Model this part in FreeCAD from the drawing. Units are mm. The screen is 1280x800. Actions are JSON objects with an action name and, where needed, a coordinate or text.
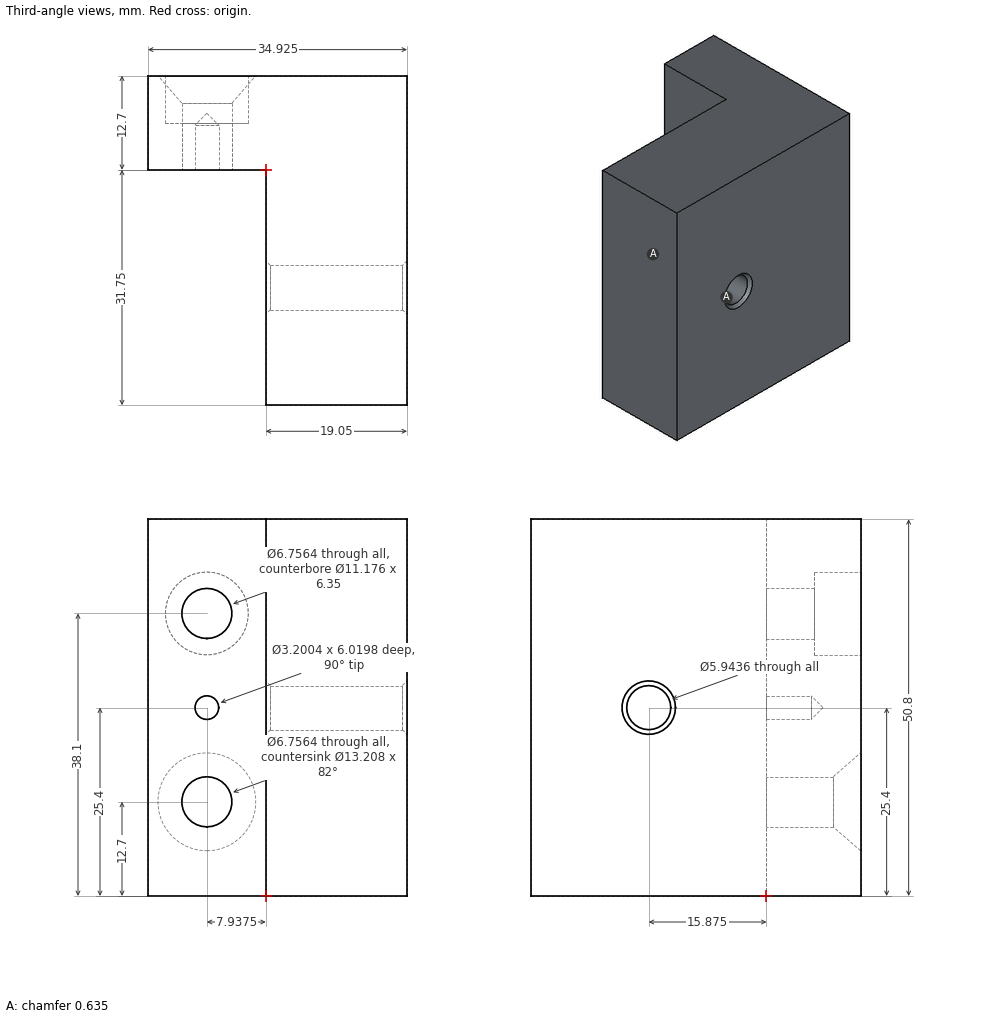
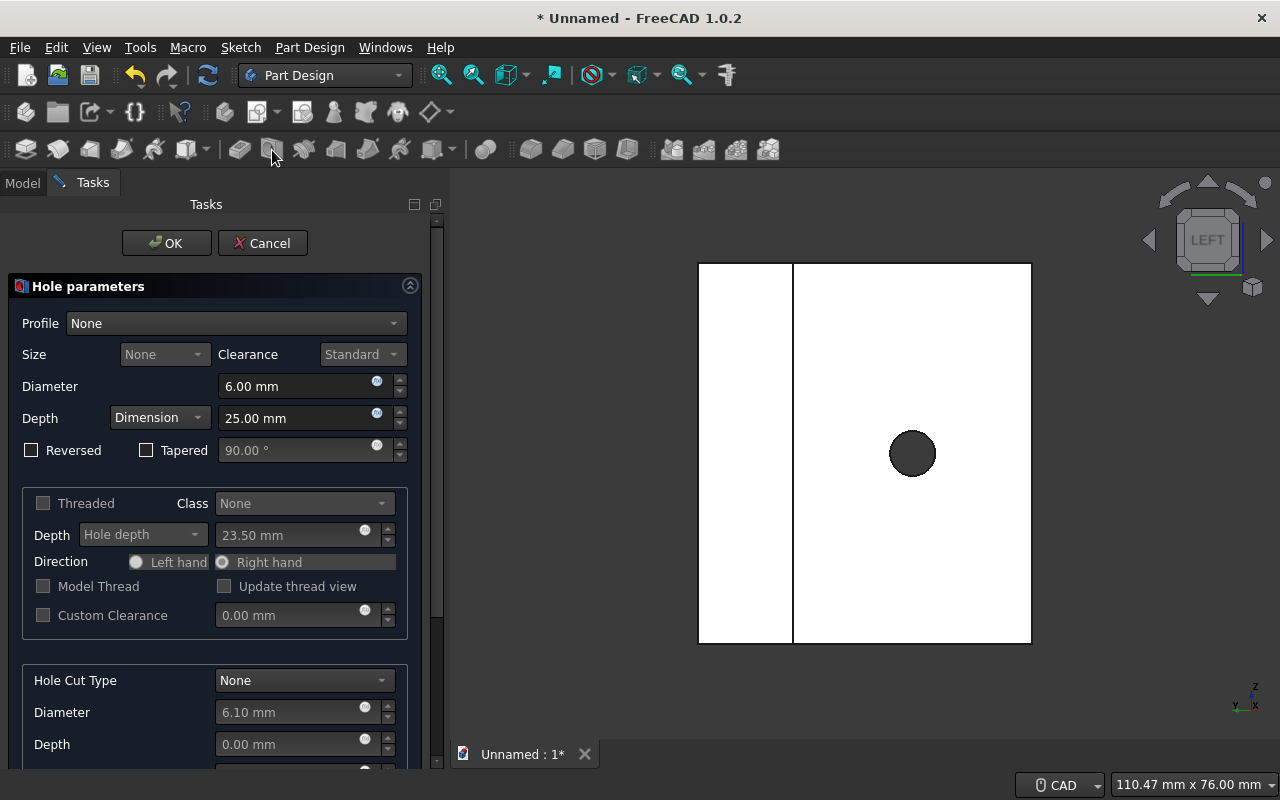
{"action": "triple_click", "coordinate": [305, 386]}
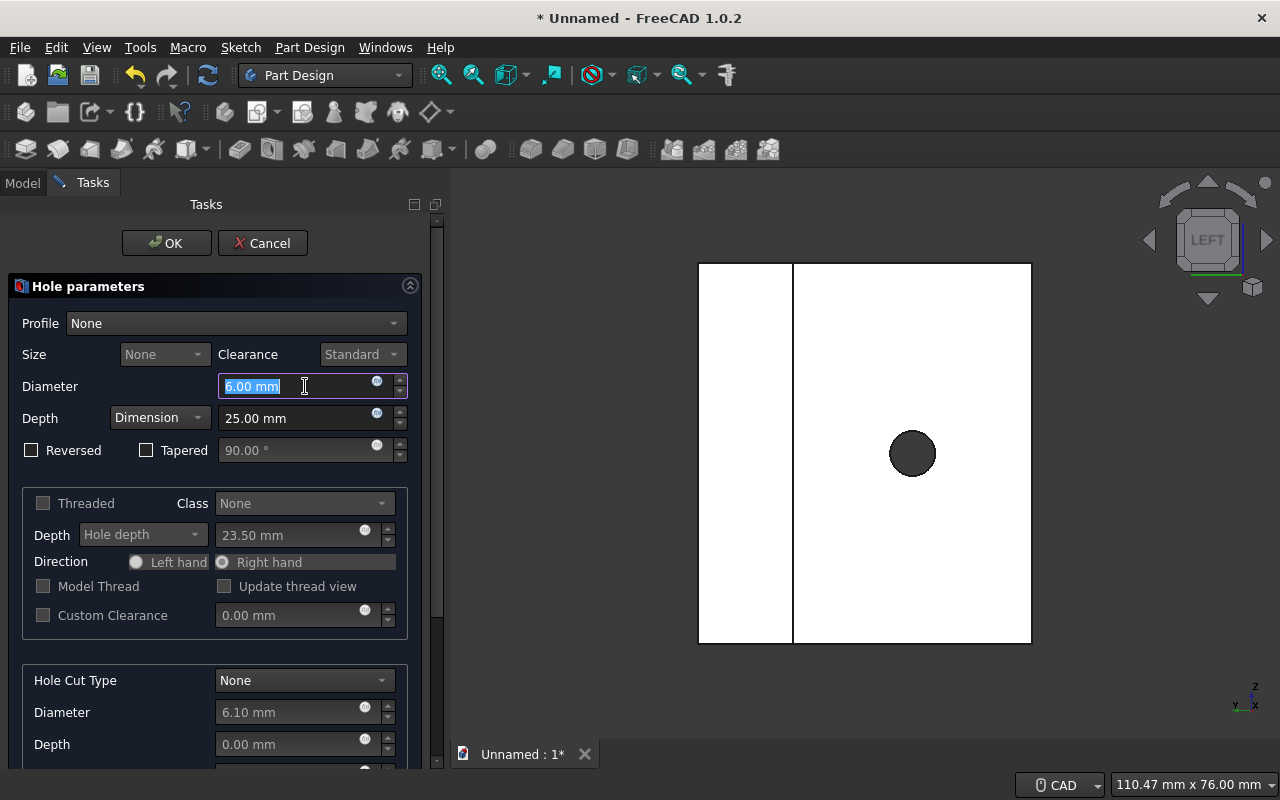
{"action": "type", "text": "5.9436"}
{"action": "key", "text": "Tab"}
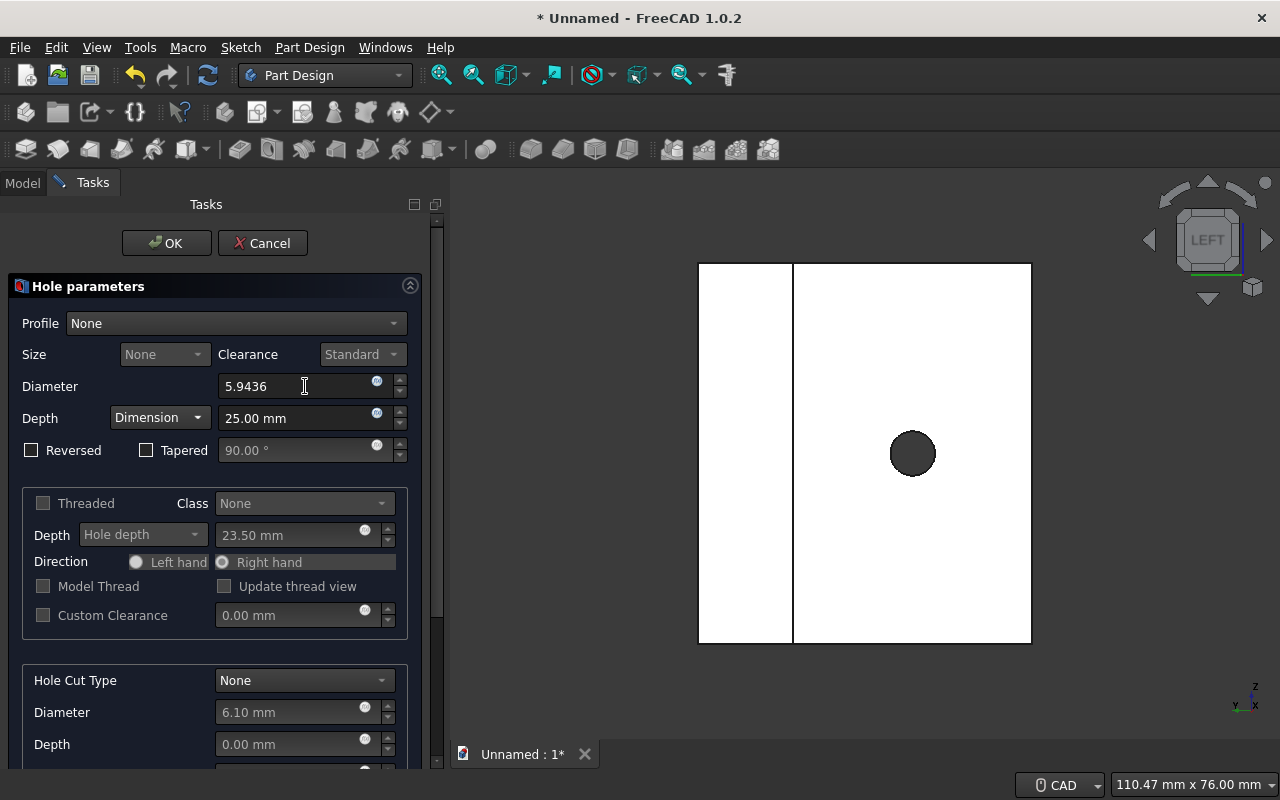
{"action": "left_click", "coordinate": [161, 418]}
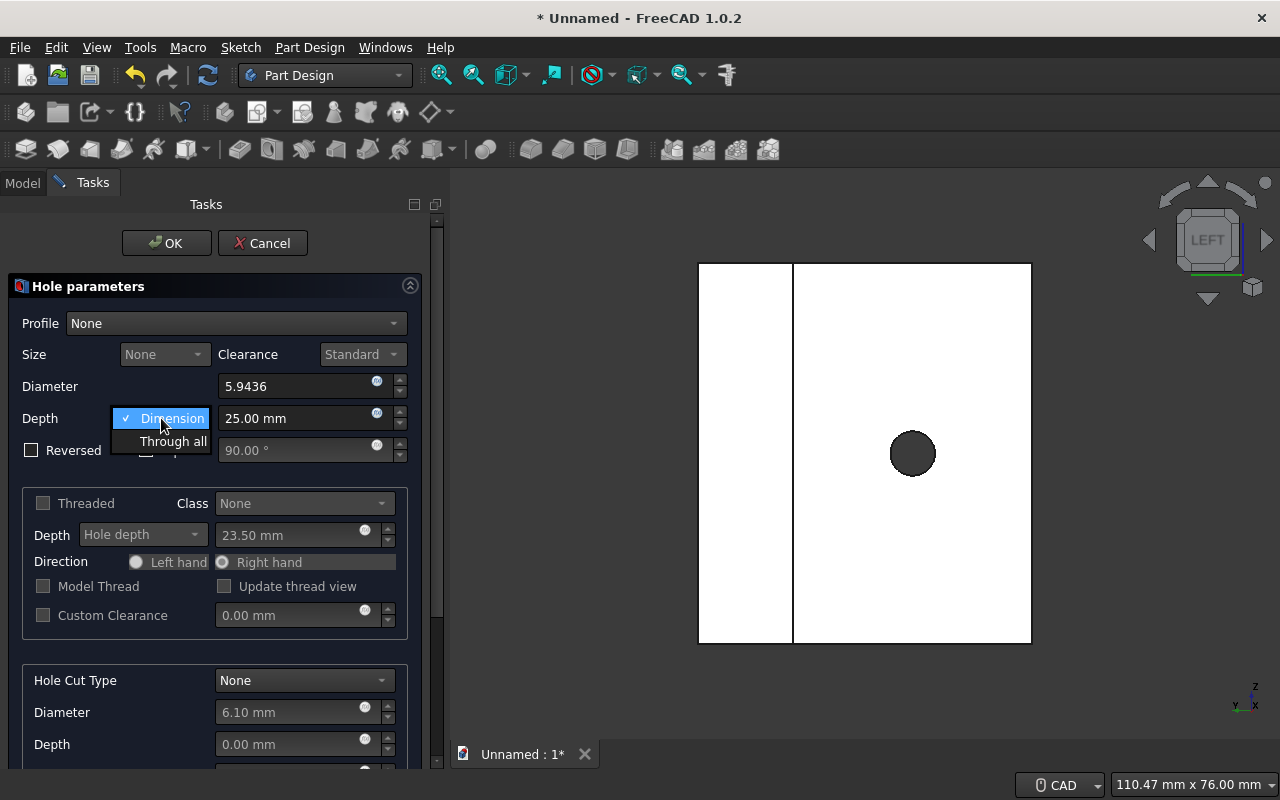
{"action": "left_click", "coordinate": [160, 442]}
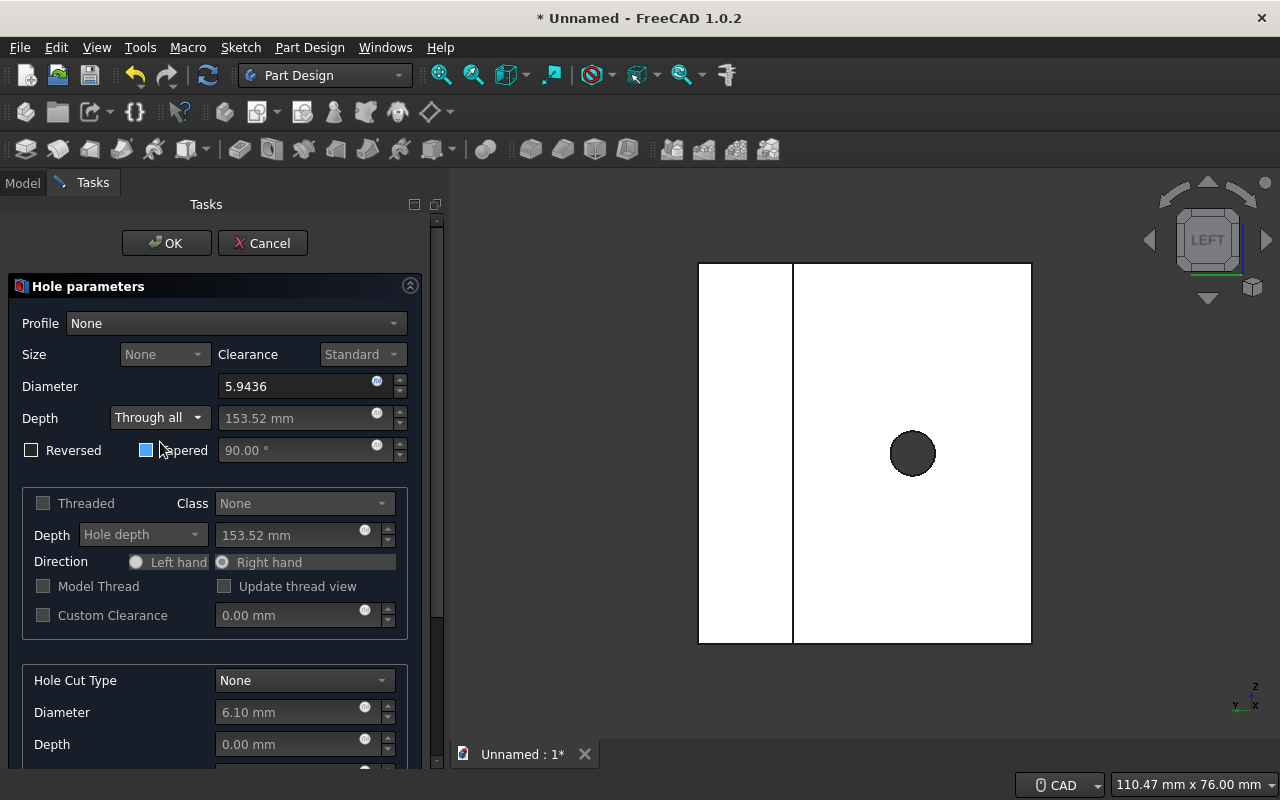
{"action": "left_click", "coordinate": [167, 243]}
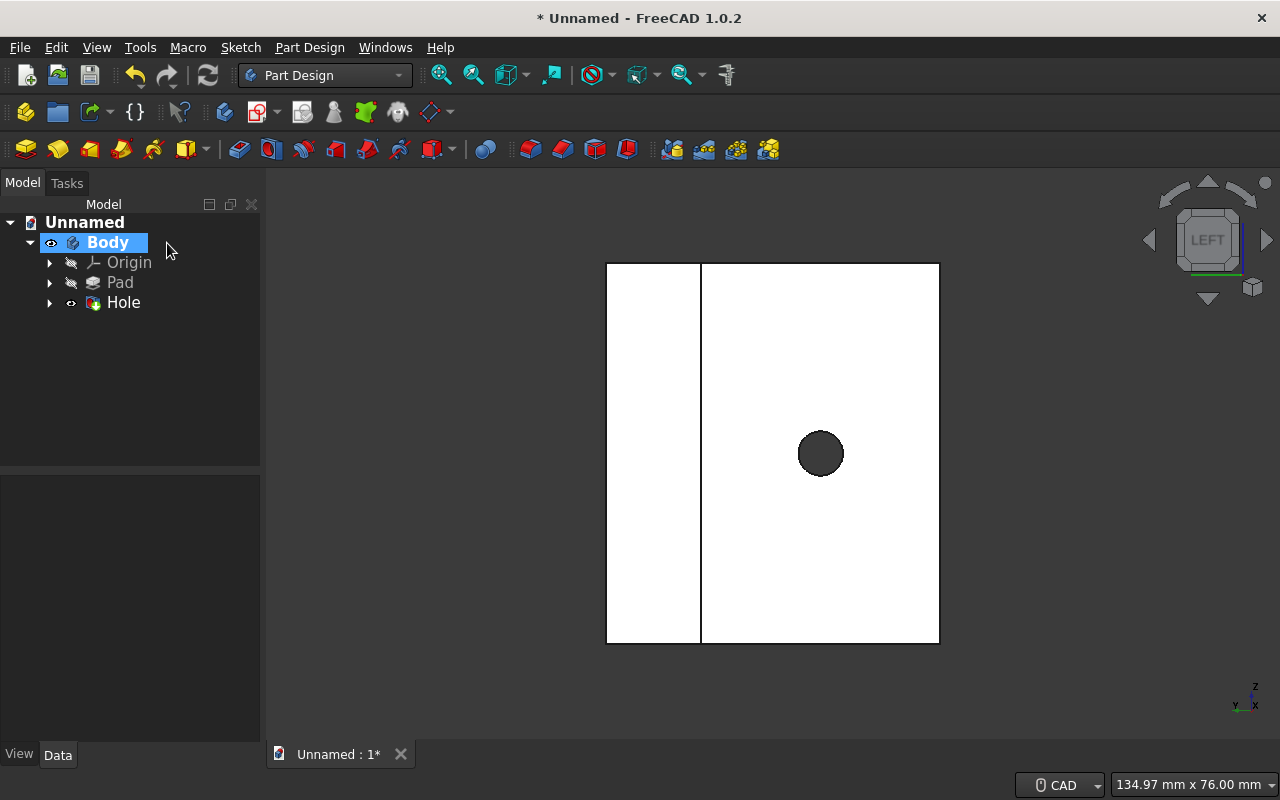
{"action": "left_click", "coordinate": [808, 471]}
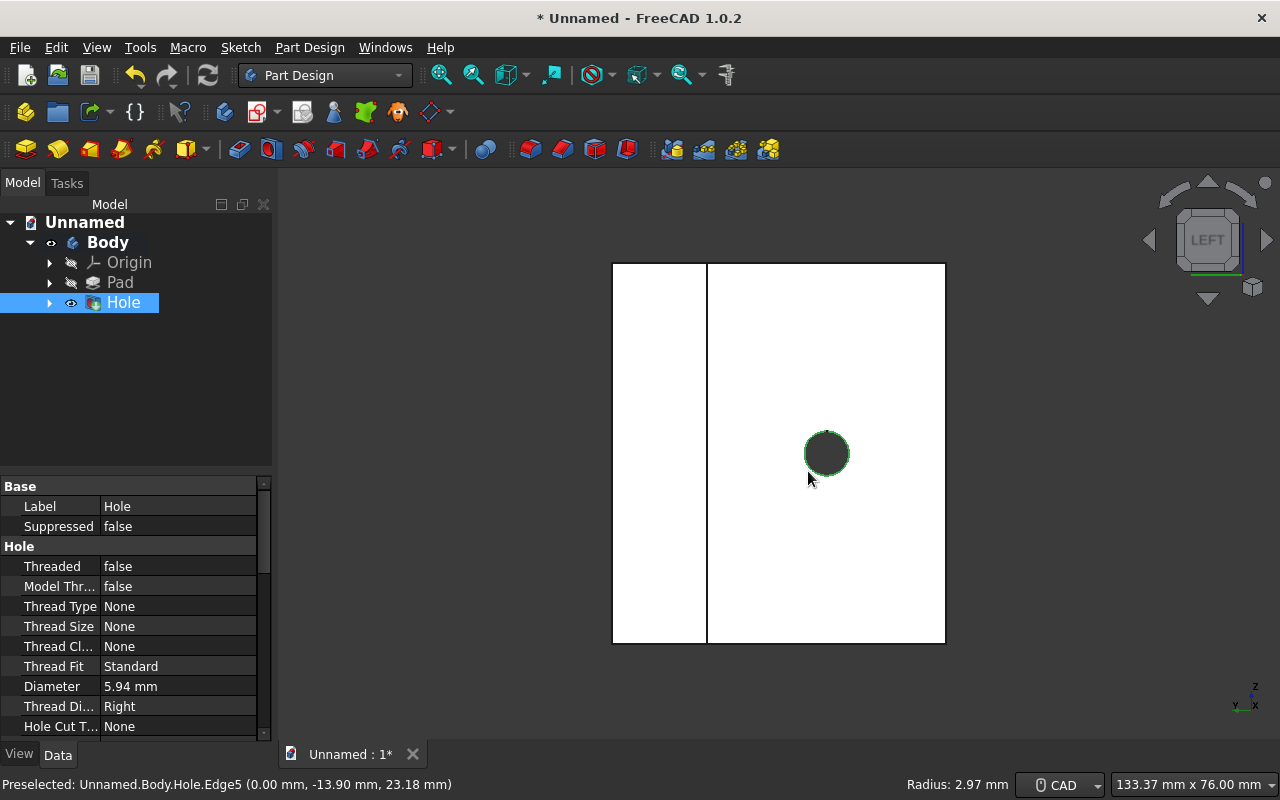
{"action": "key", "text": "0"}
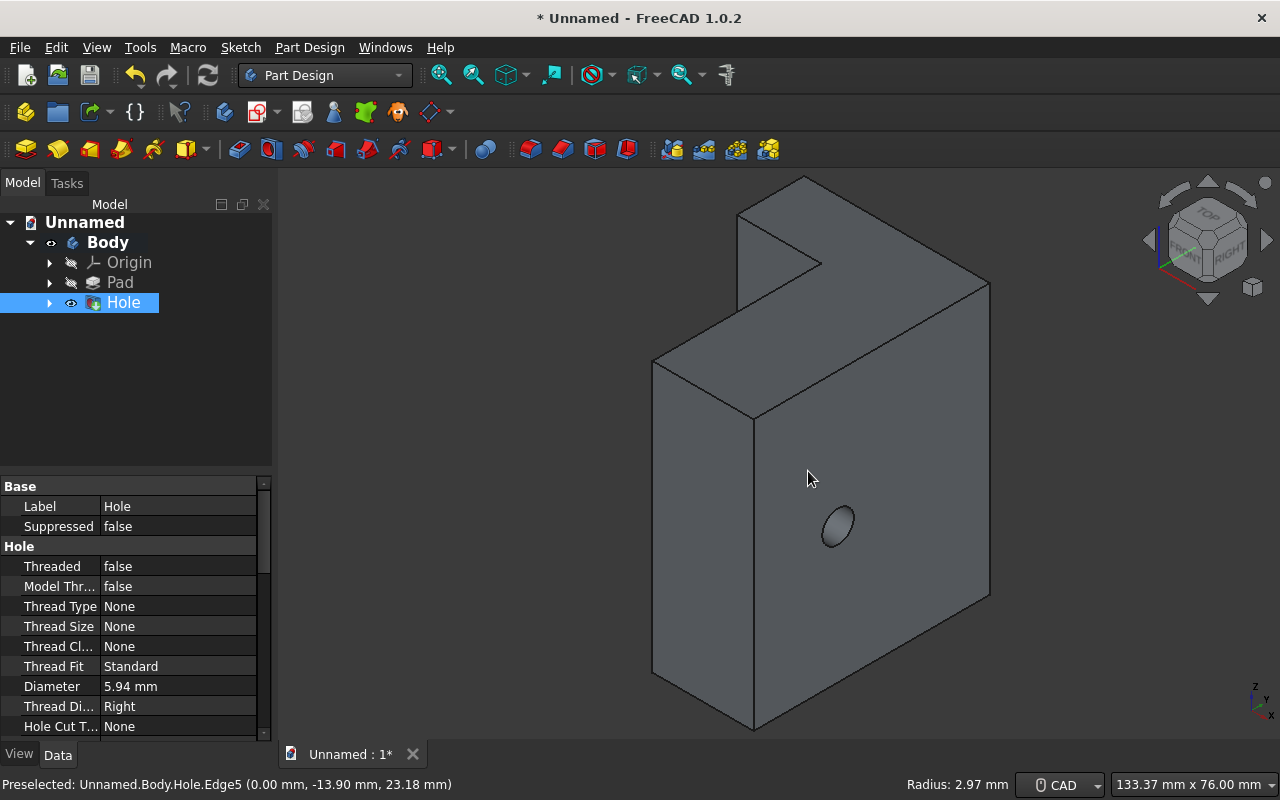
{"action": "left_click", "coordinate": [838, 544], "text": "ctrl"}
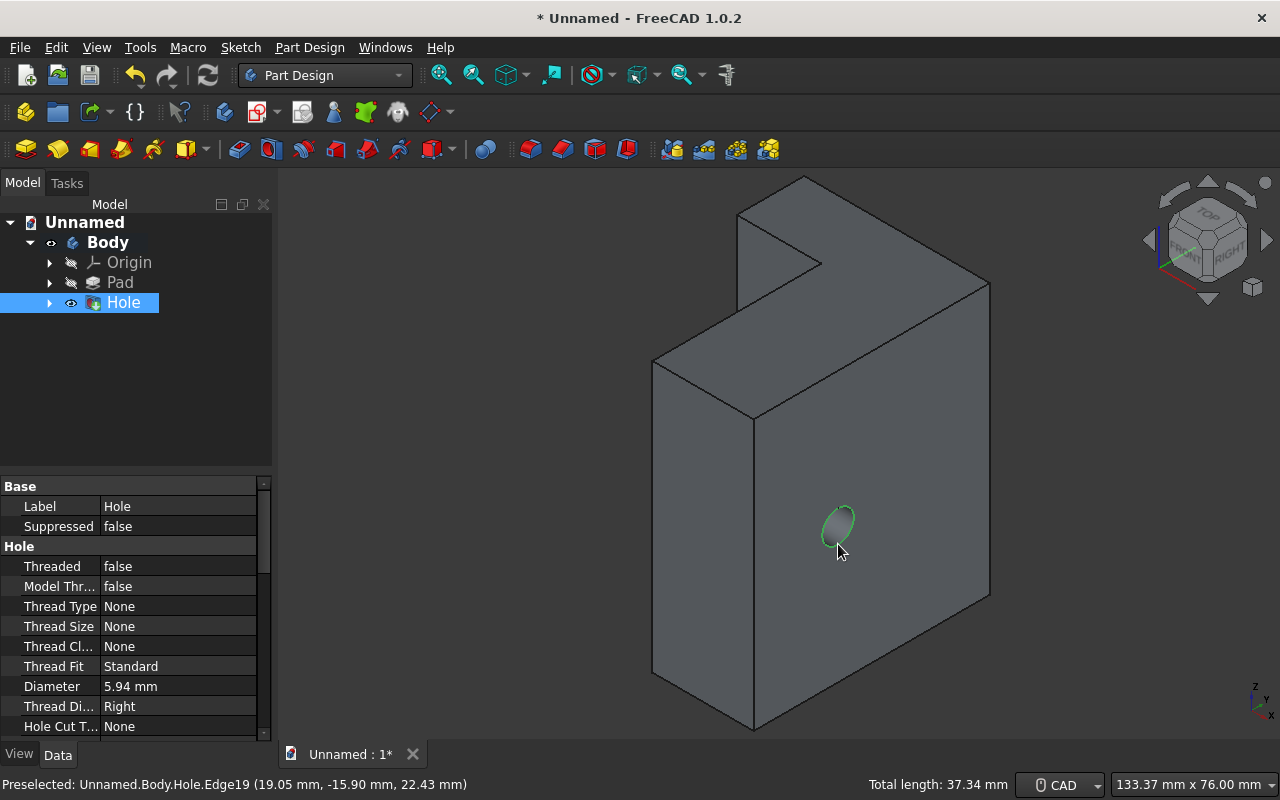
{"action": "left_click", "coordinate": [564, 150]}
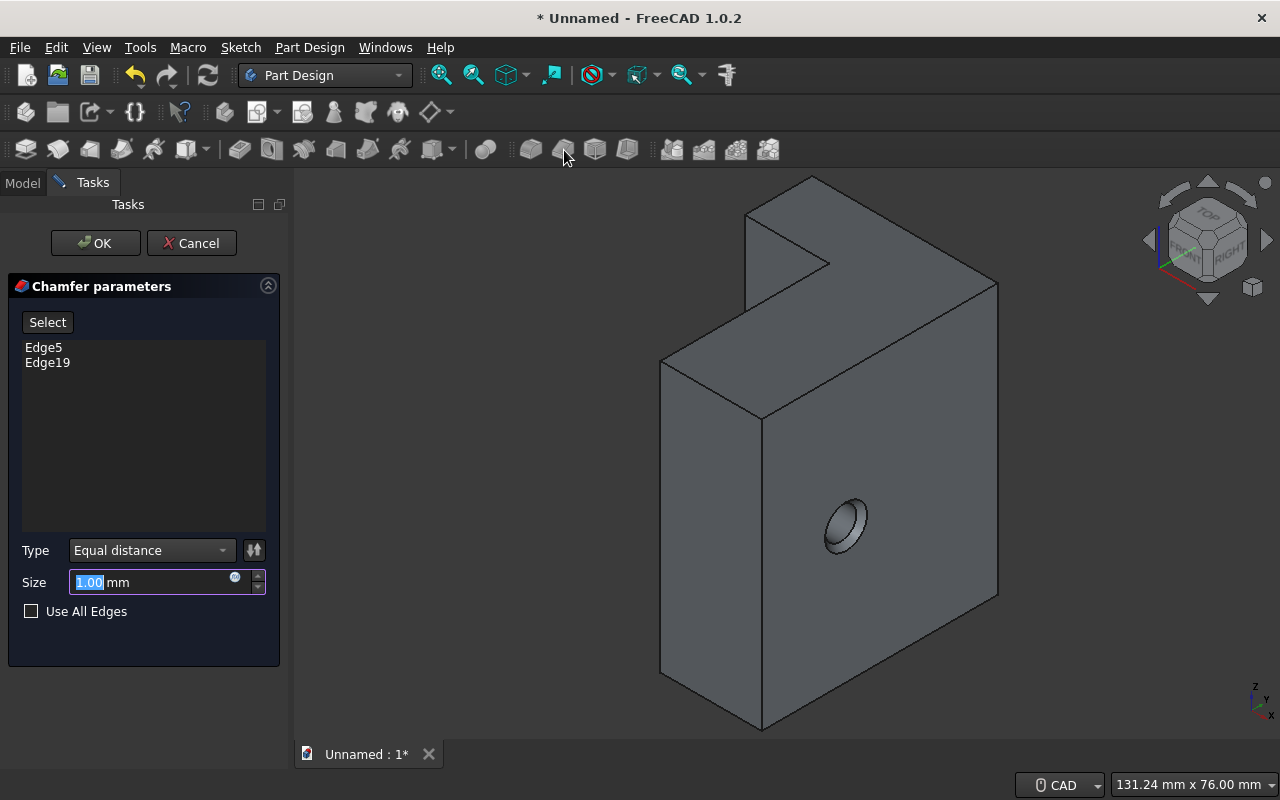
{"action": "type", "text": "0.635"}
{"action": "key", "text": "Tab"}